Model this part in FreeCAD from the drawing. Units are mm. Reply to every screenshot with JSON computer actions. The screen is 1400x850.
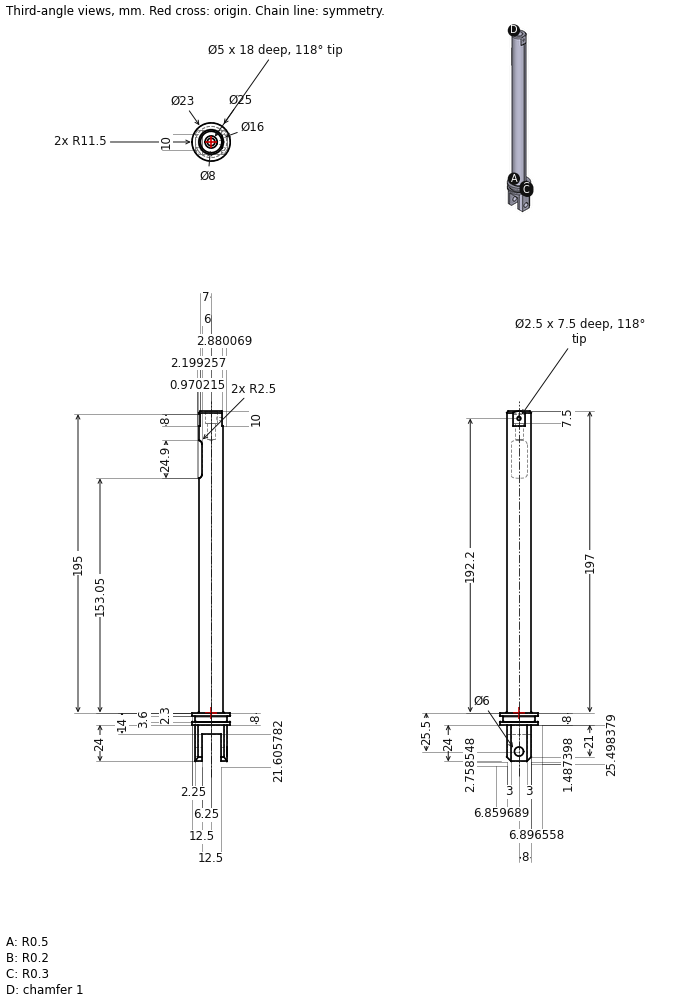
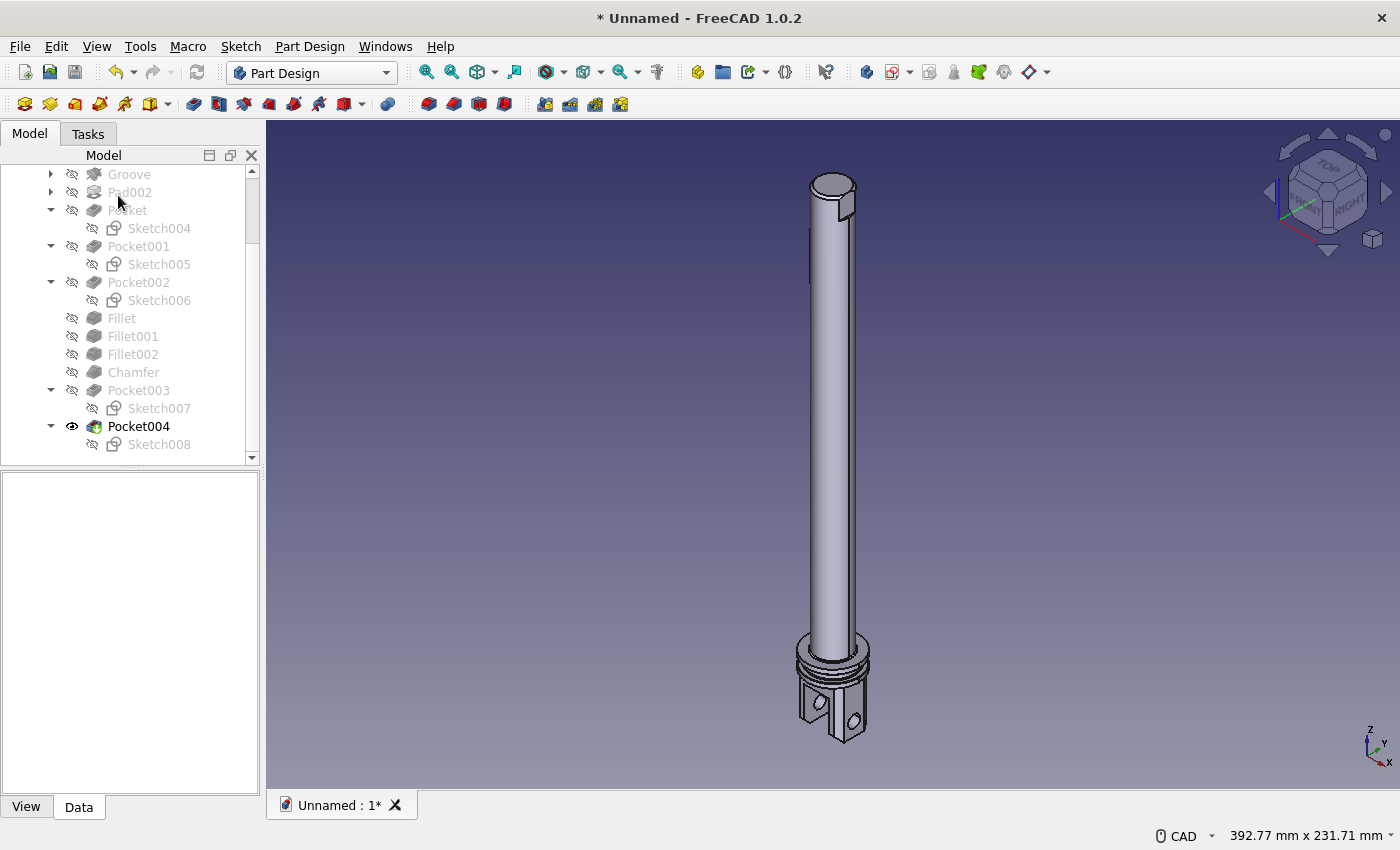
{"action": "left_click", "coordinate": [833, 184]}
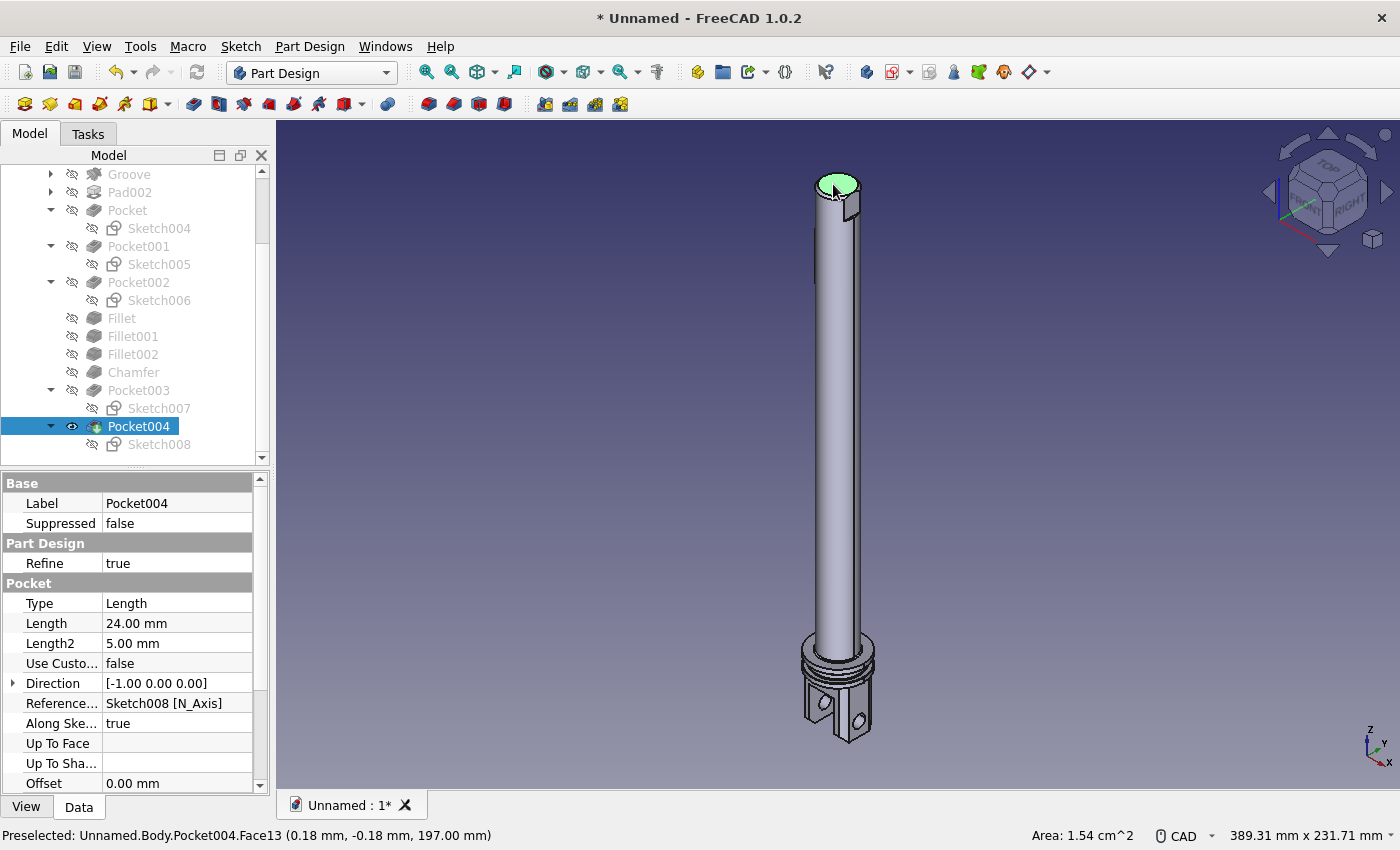
{"action": "left_click", "coordinate": [892, 72]}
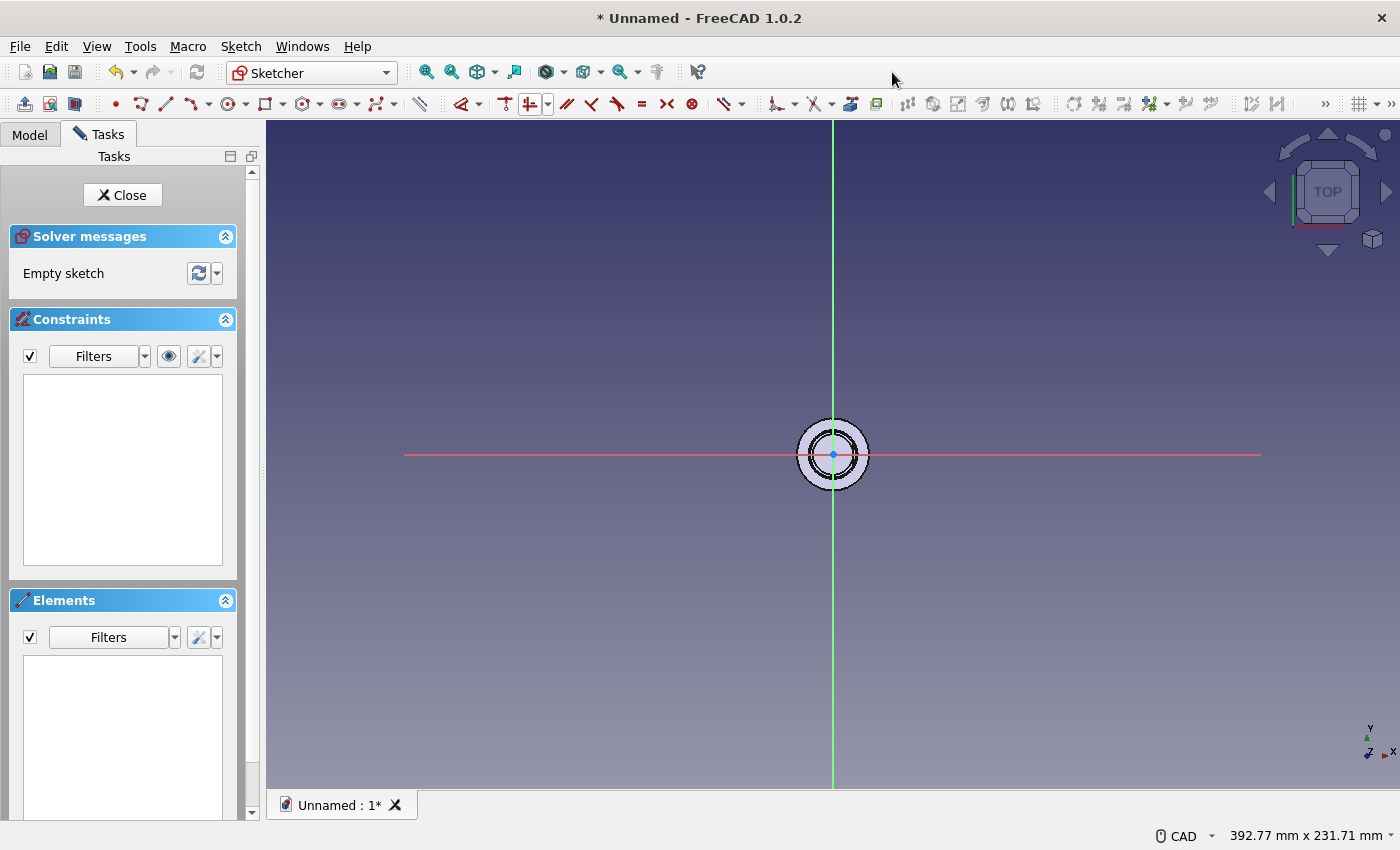
{"action": "scroll", "coordinate": [837, 454], "scroll_direction": "up", "scroll_amount": 15}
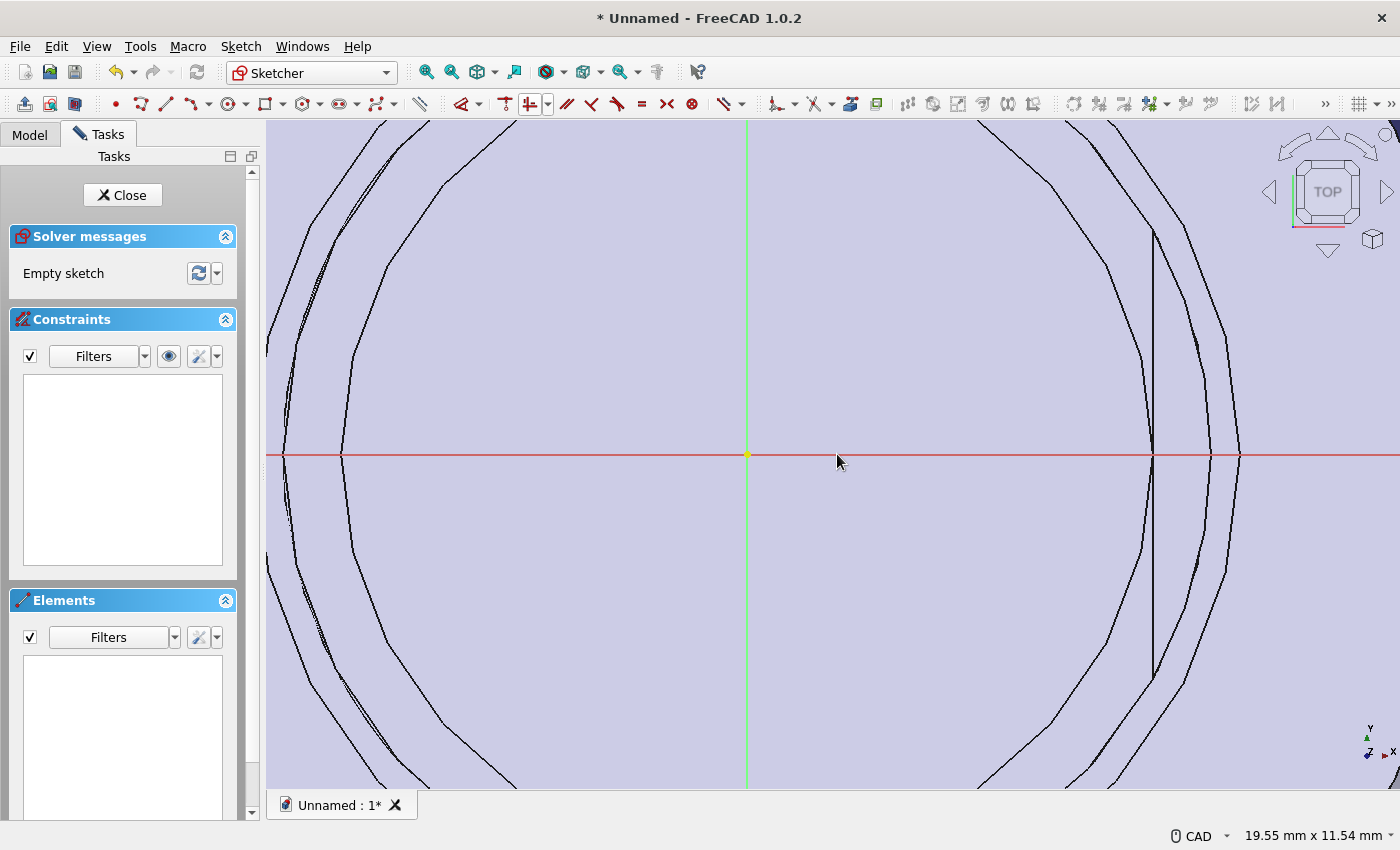
{"action": "left_click", "coordinate": [228, 104]}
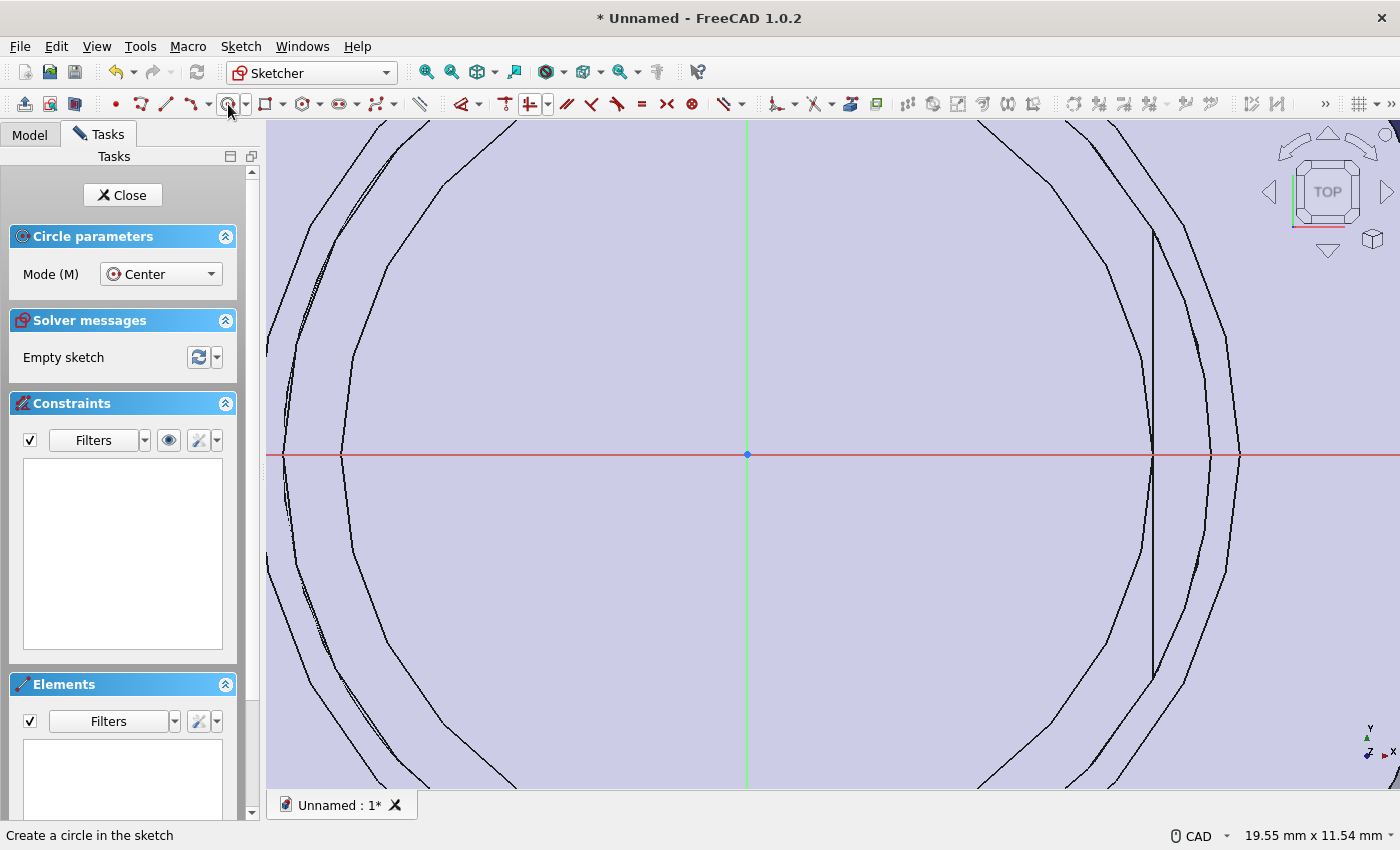
{"action": "left_click", "coordinate": [747, 454]}
{"action": "mouse_move", "coordinate": [911, 290]}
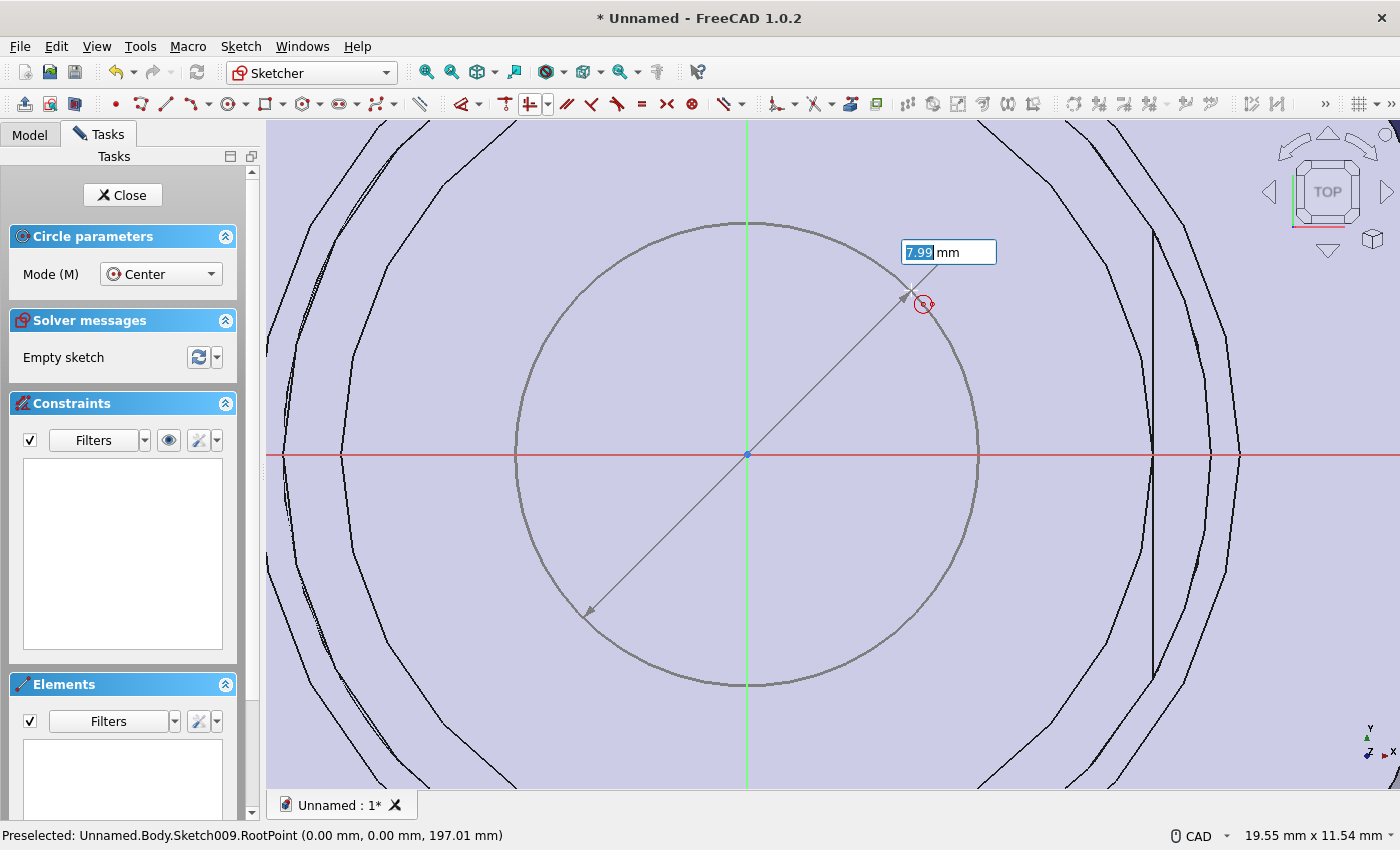
{"action": "type", "text": "8"}
{"action": "key", "text": "Return"}
{"action": "key", "text": "Escape"}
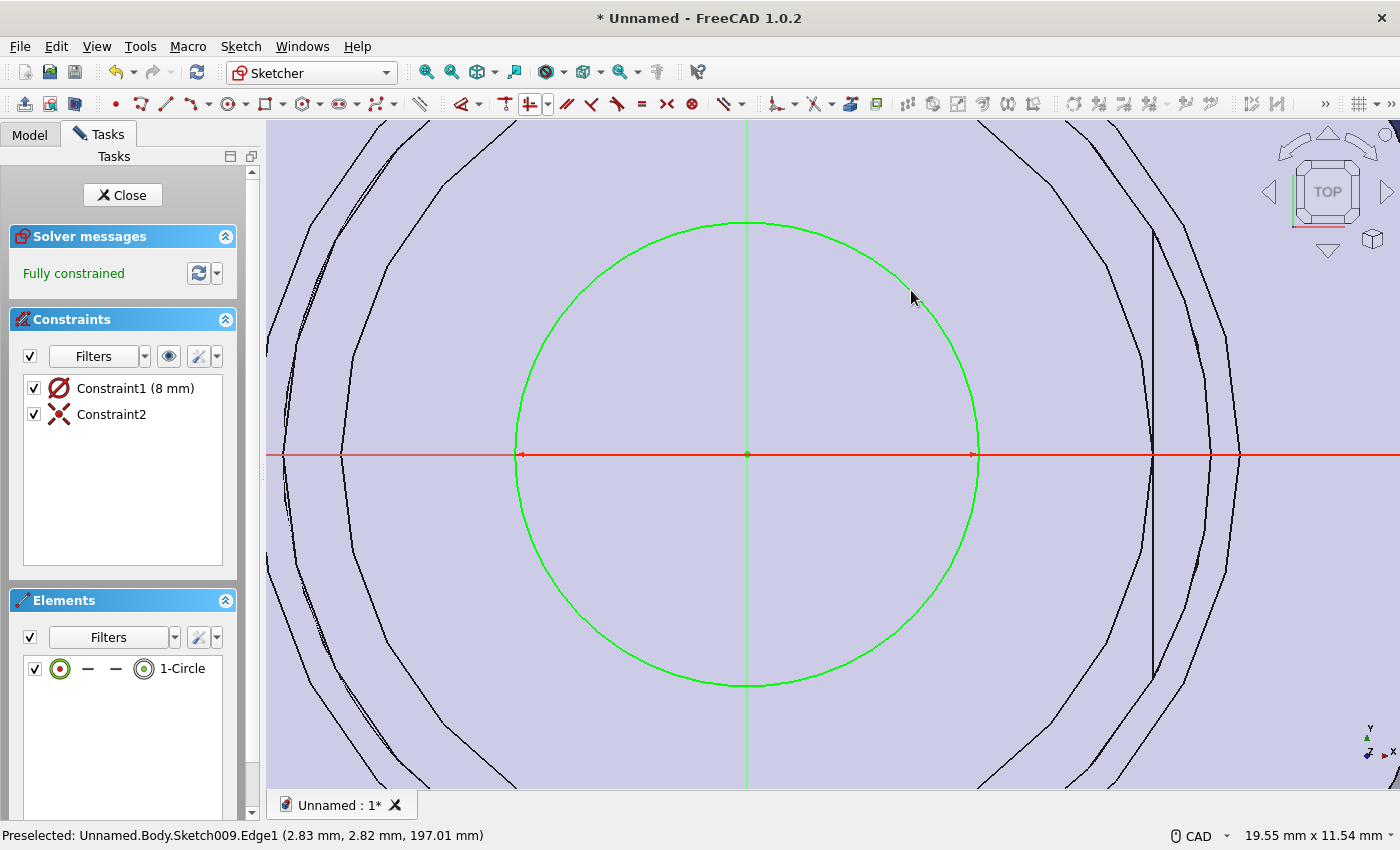
{"action": "left_click", "coordinate": [123, 195]}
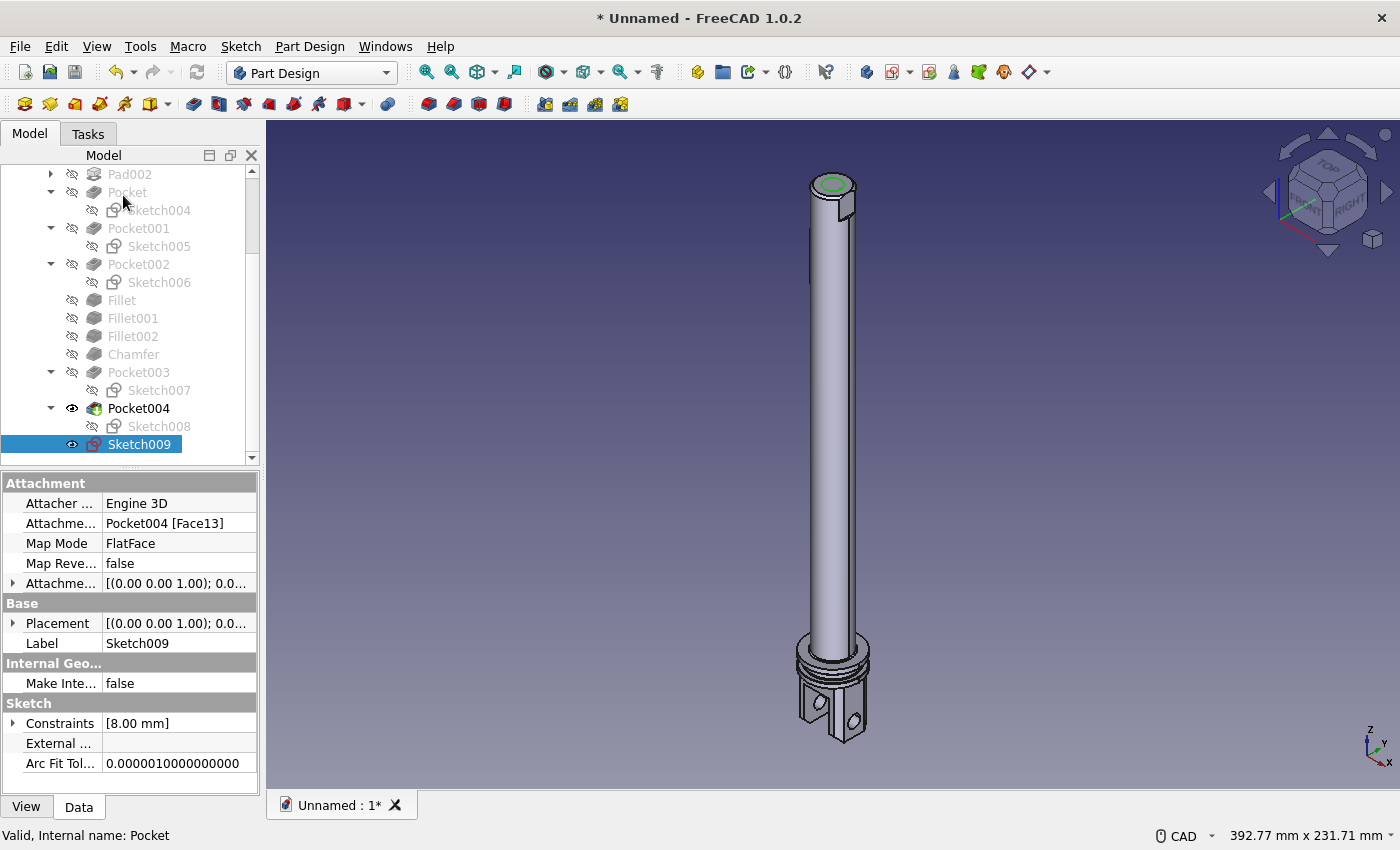
{"action": "left_click", "coordinate": [194, 104]}